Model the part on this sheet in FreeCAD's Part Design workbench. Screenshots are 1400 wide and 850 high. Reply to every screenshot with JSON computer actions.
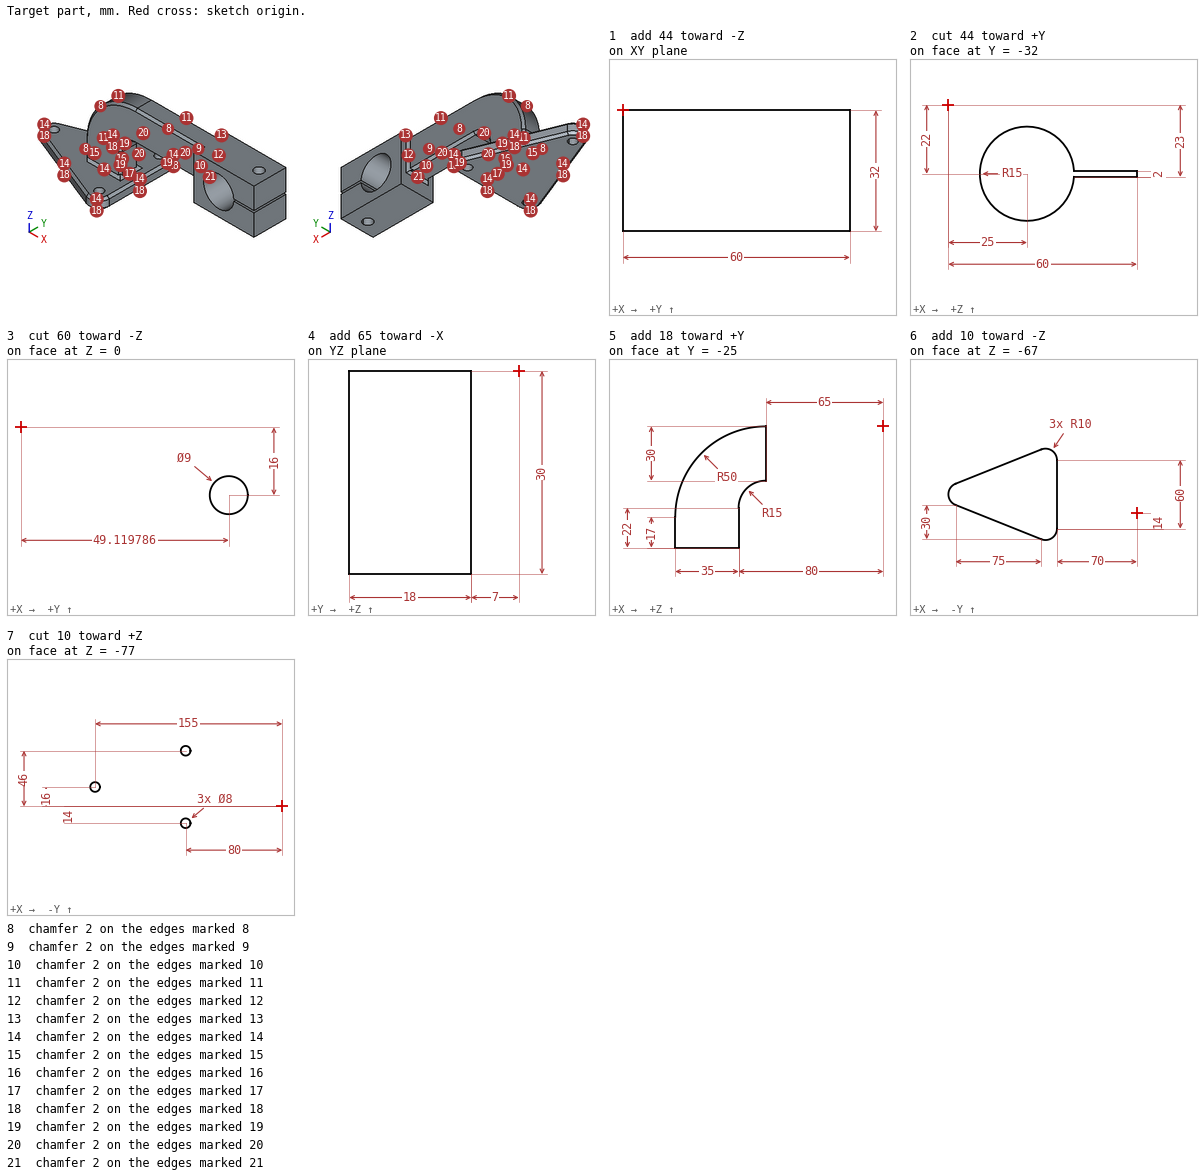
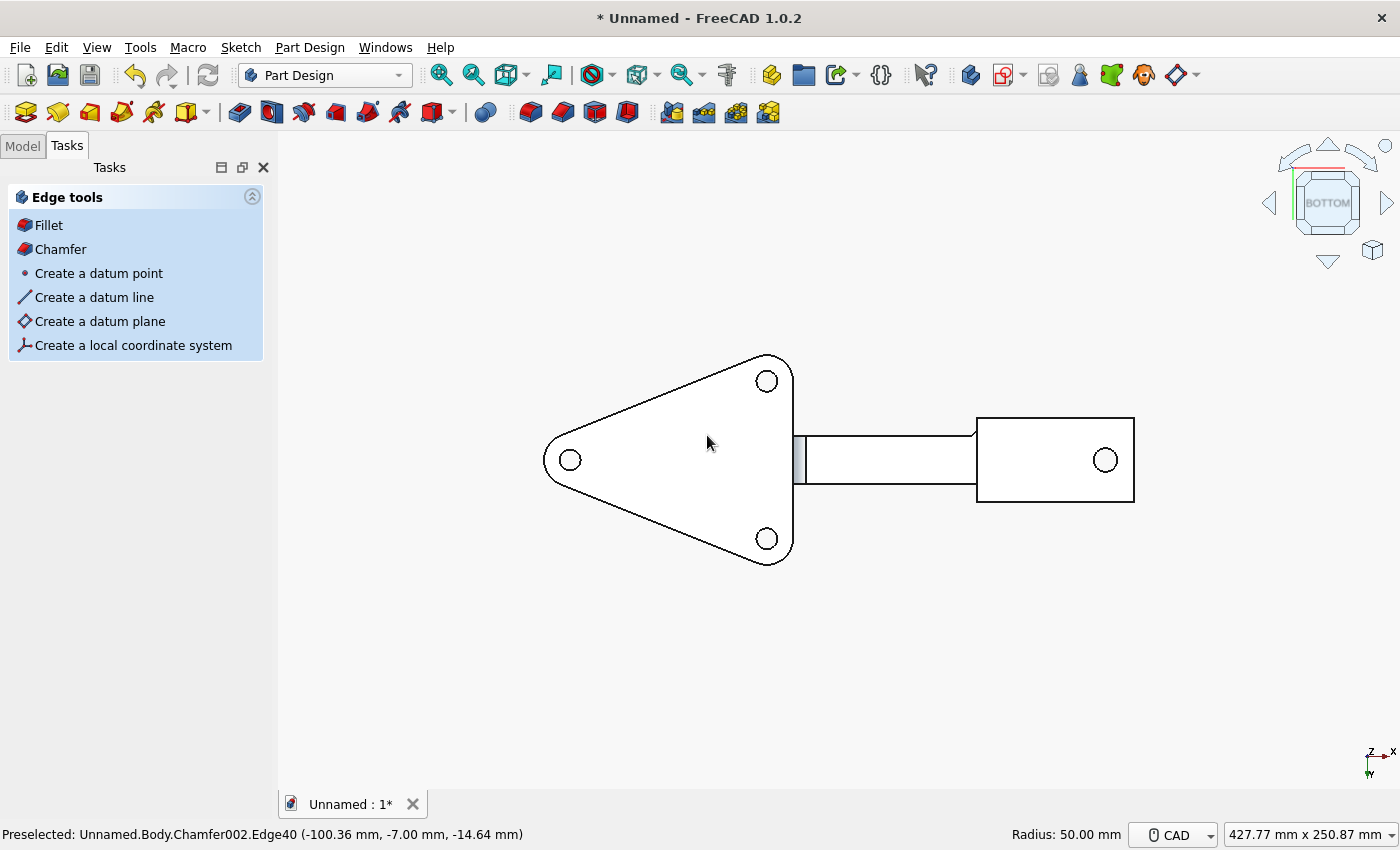
{"action": "key", "text": "4"}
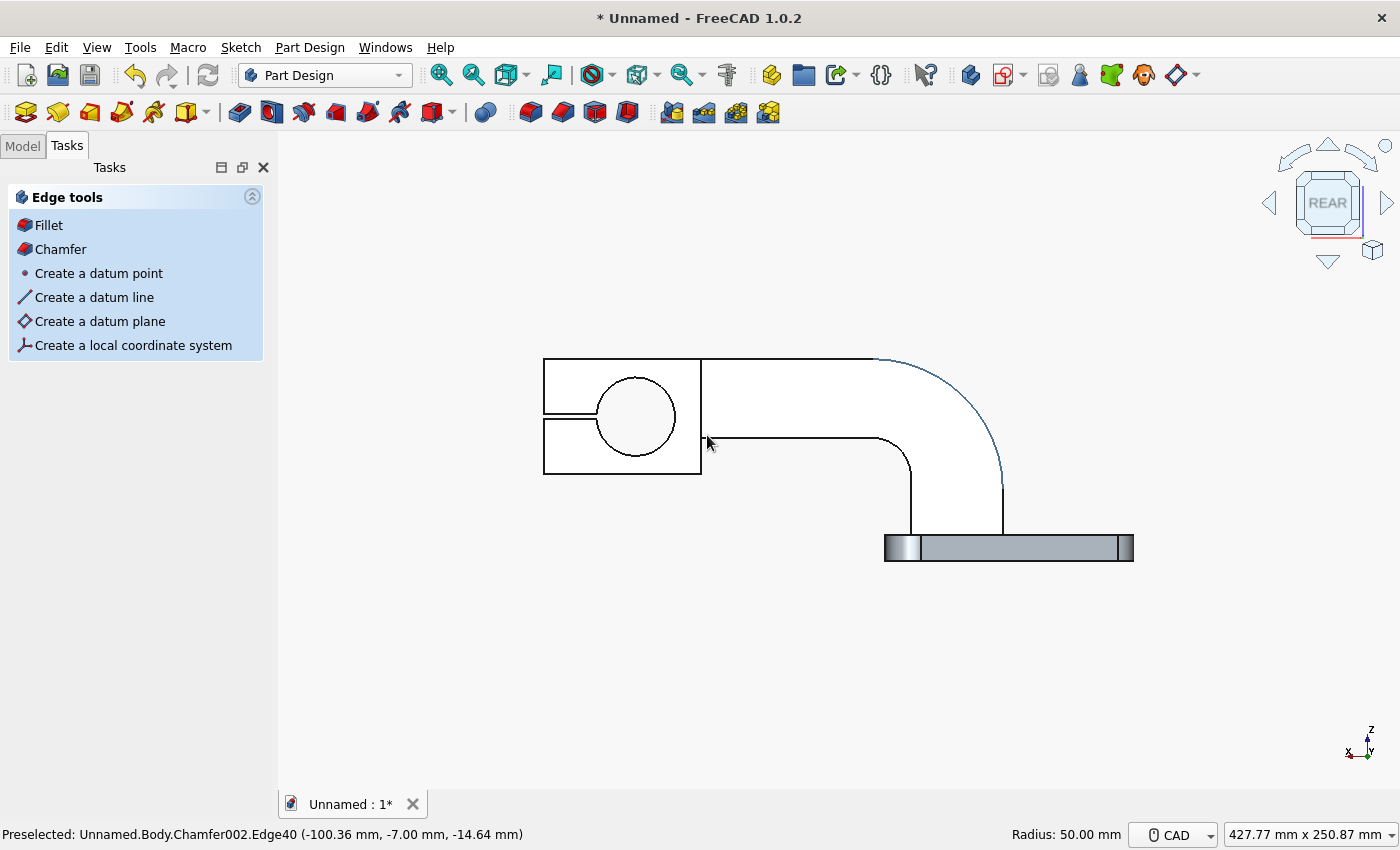
{"action": "left_click", "coordinate": [787, 358], "text": "ctrl"}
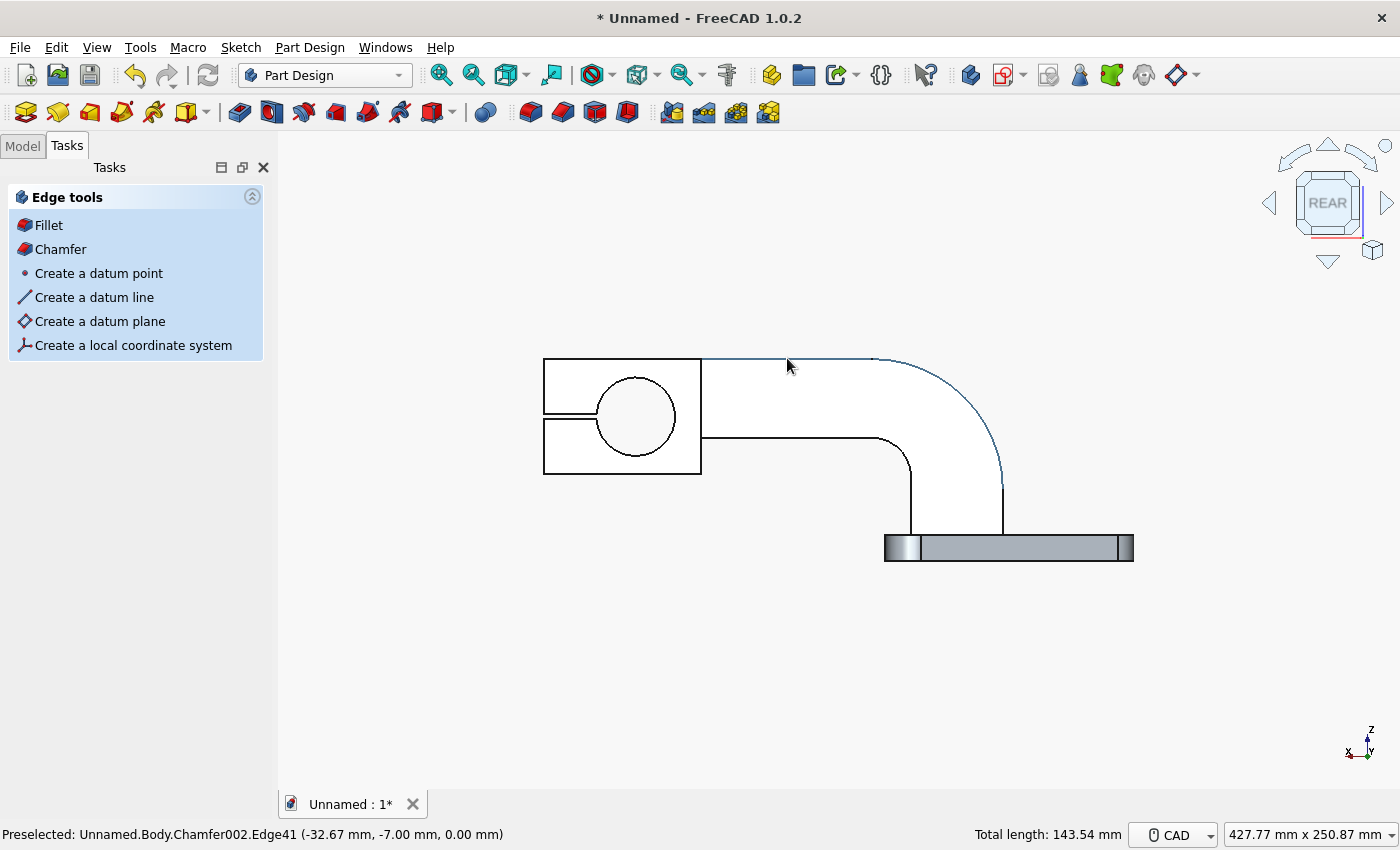
{"action": "left_click", "coordinate": [1003, 511], "text": "ctrl"}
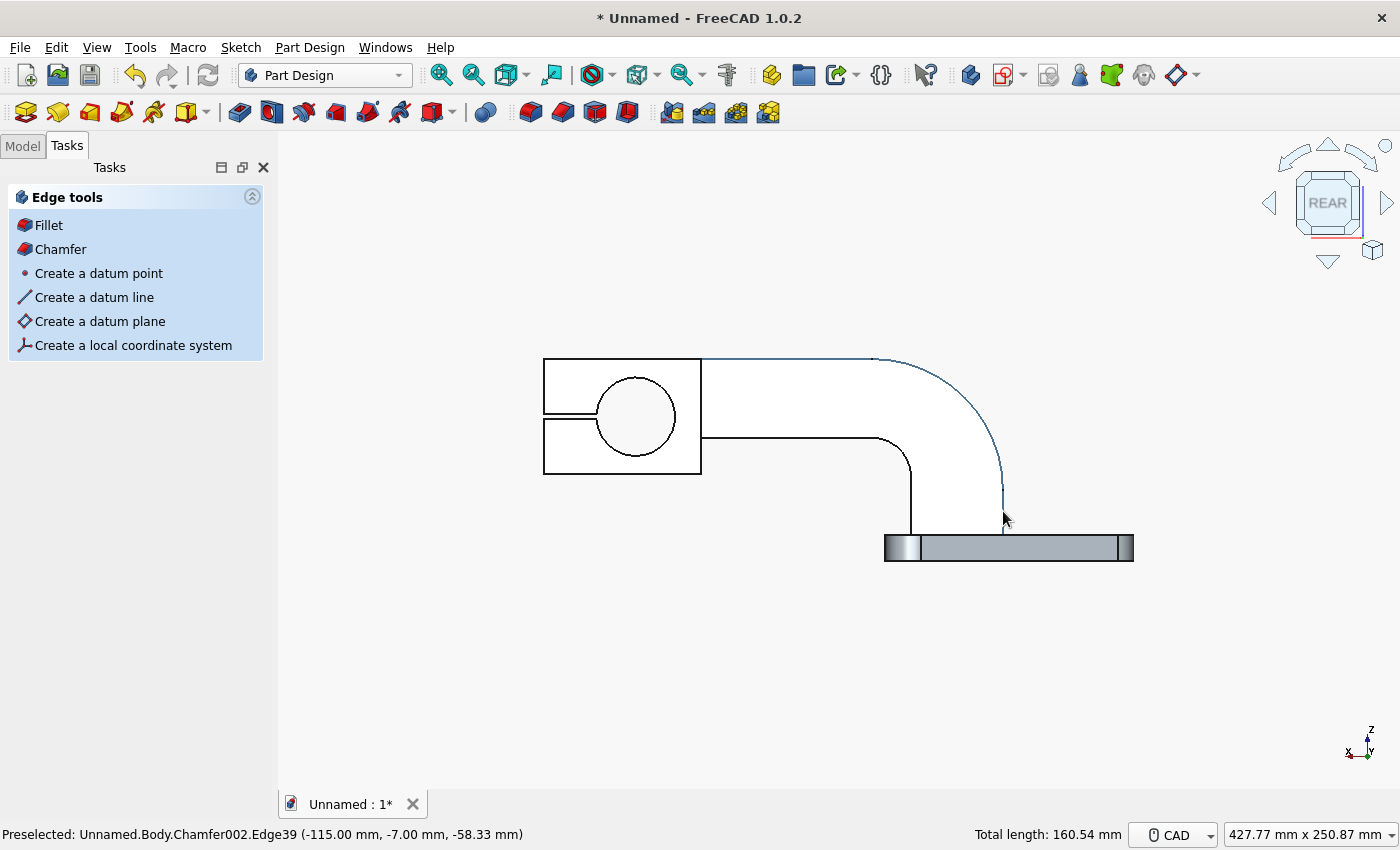
{"action": "left_click", "coordinate": [564, 112]}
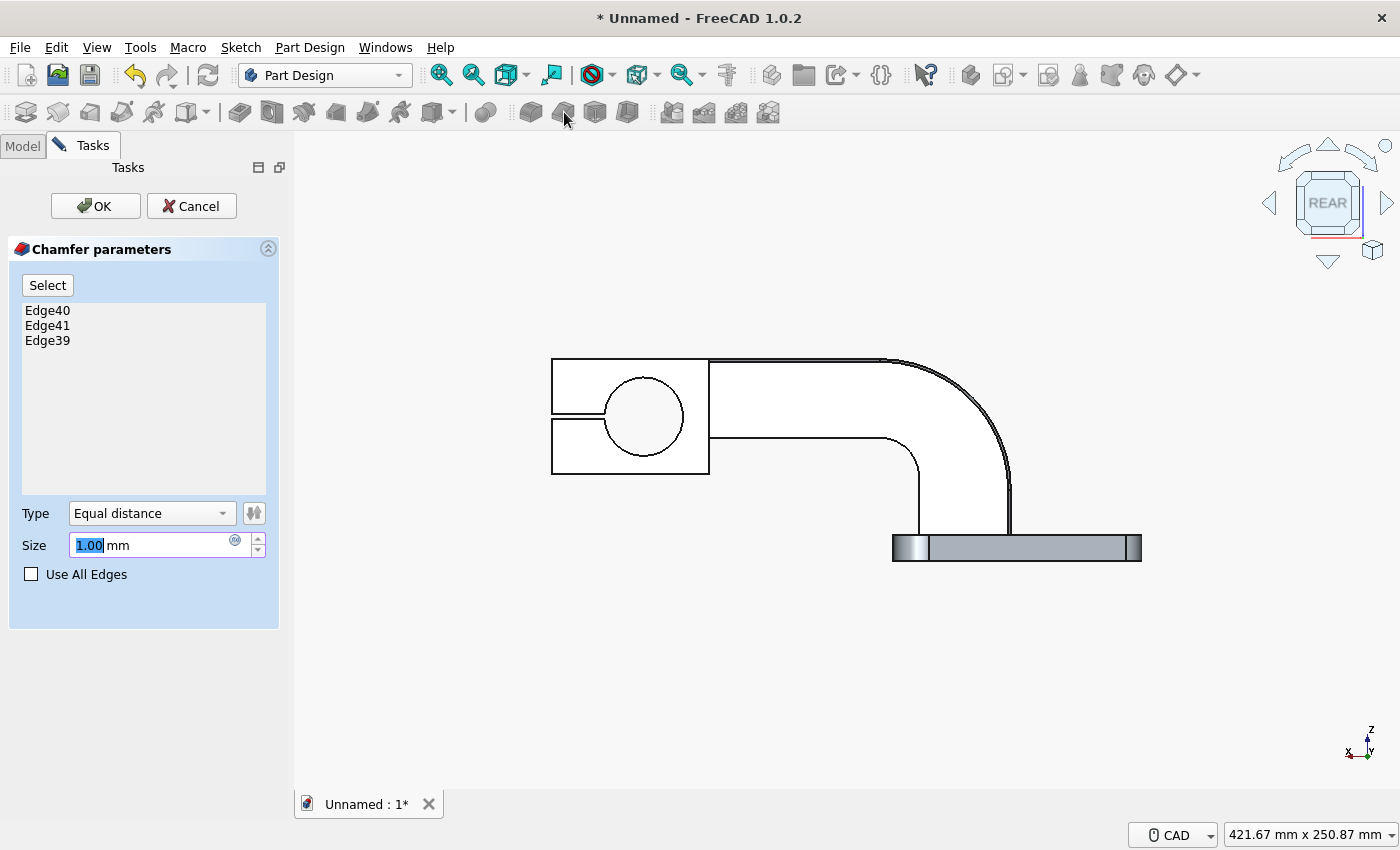
{"action": "type", "text": "2"}
{"action": "key", "text": "Tab"}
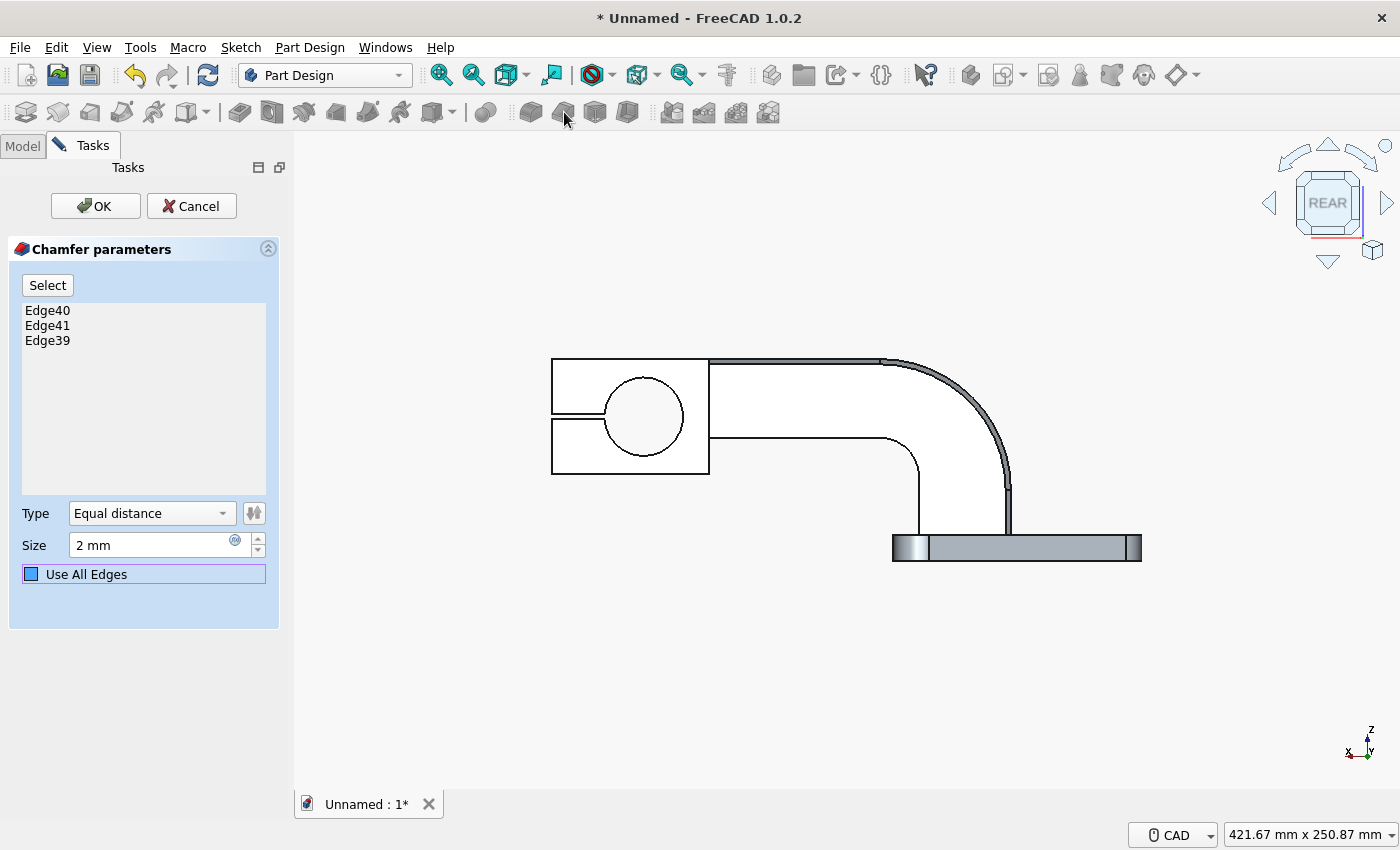
{"action": "left_click", "coordinate": [96, 206]}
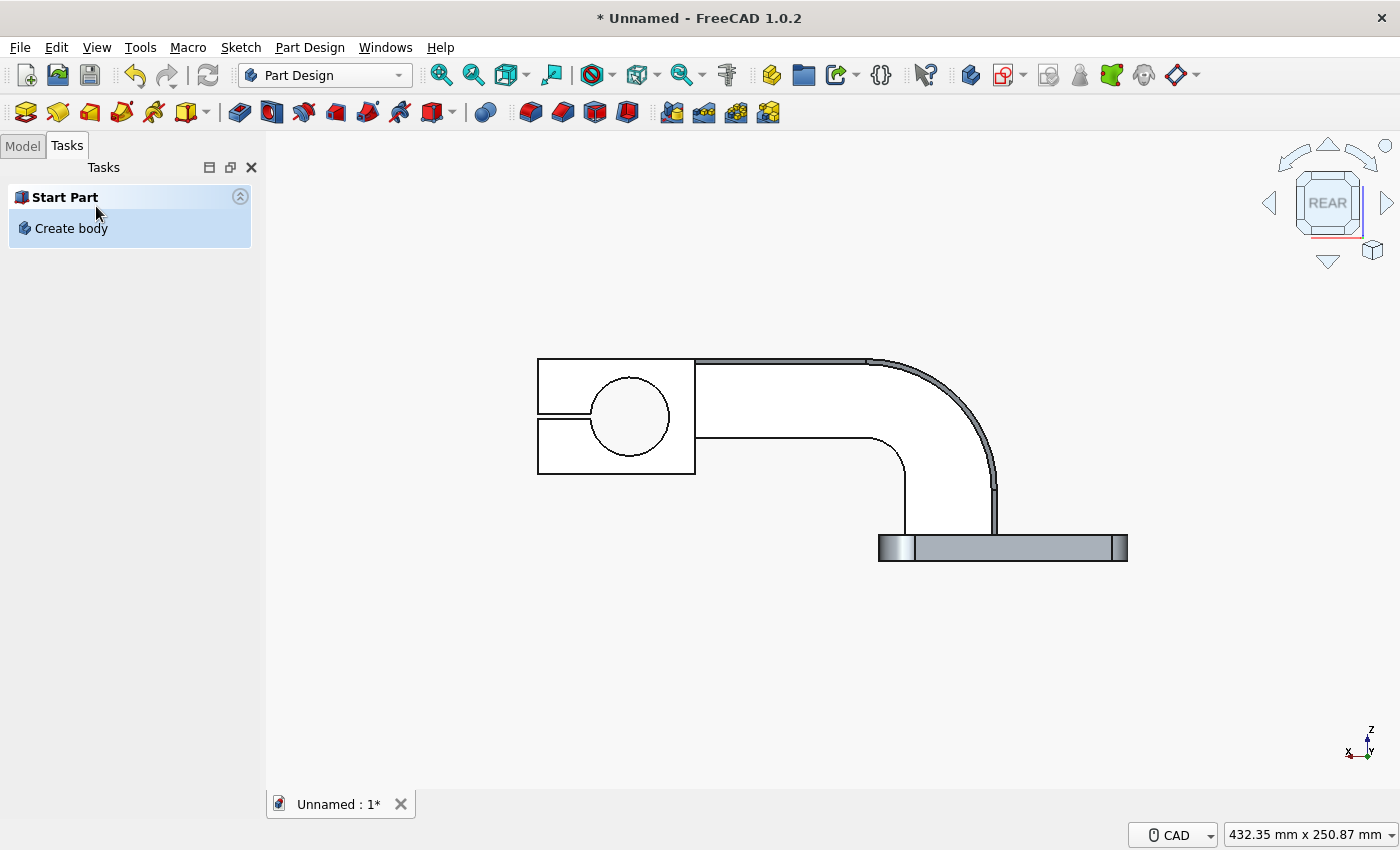
{"action": "key", "text": "0"}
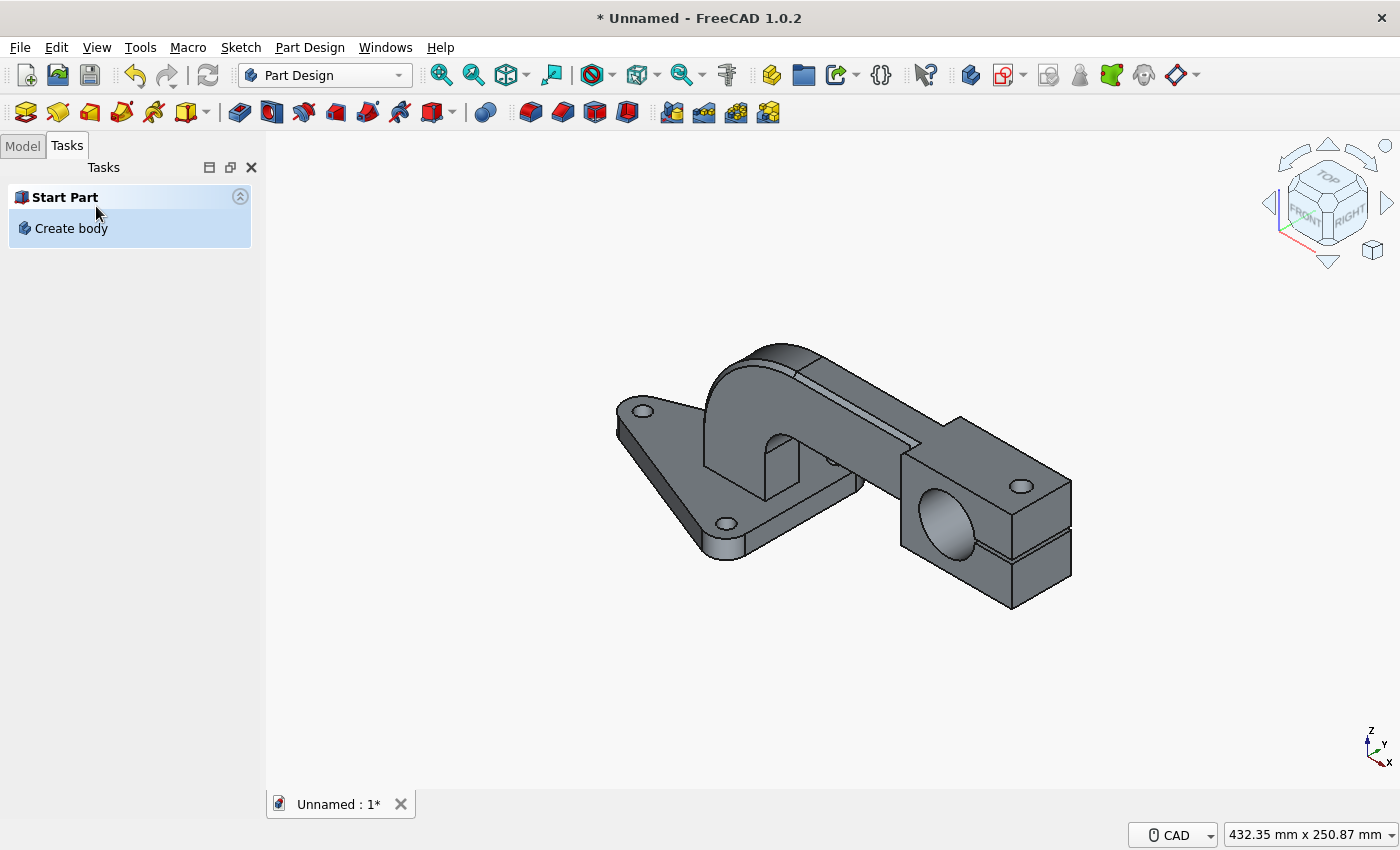
{"action": "key", "text": "2"}